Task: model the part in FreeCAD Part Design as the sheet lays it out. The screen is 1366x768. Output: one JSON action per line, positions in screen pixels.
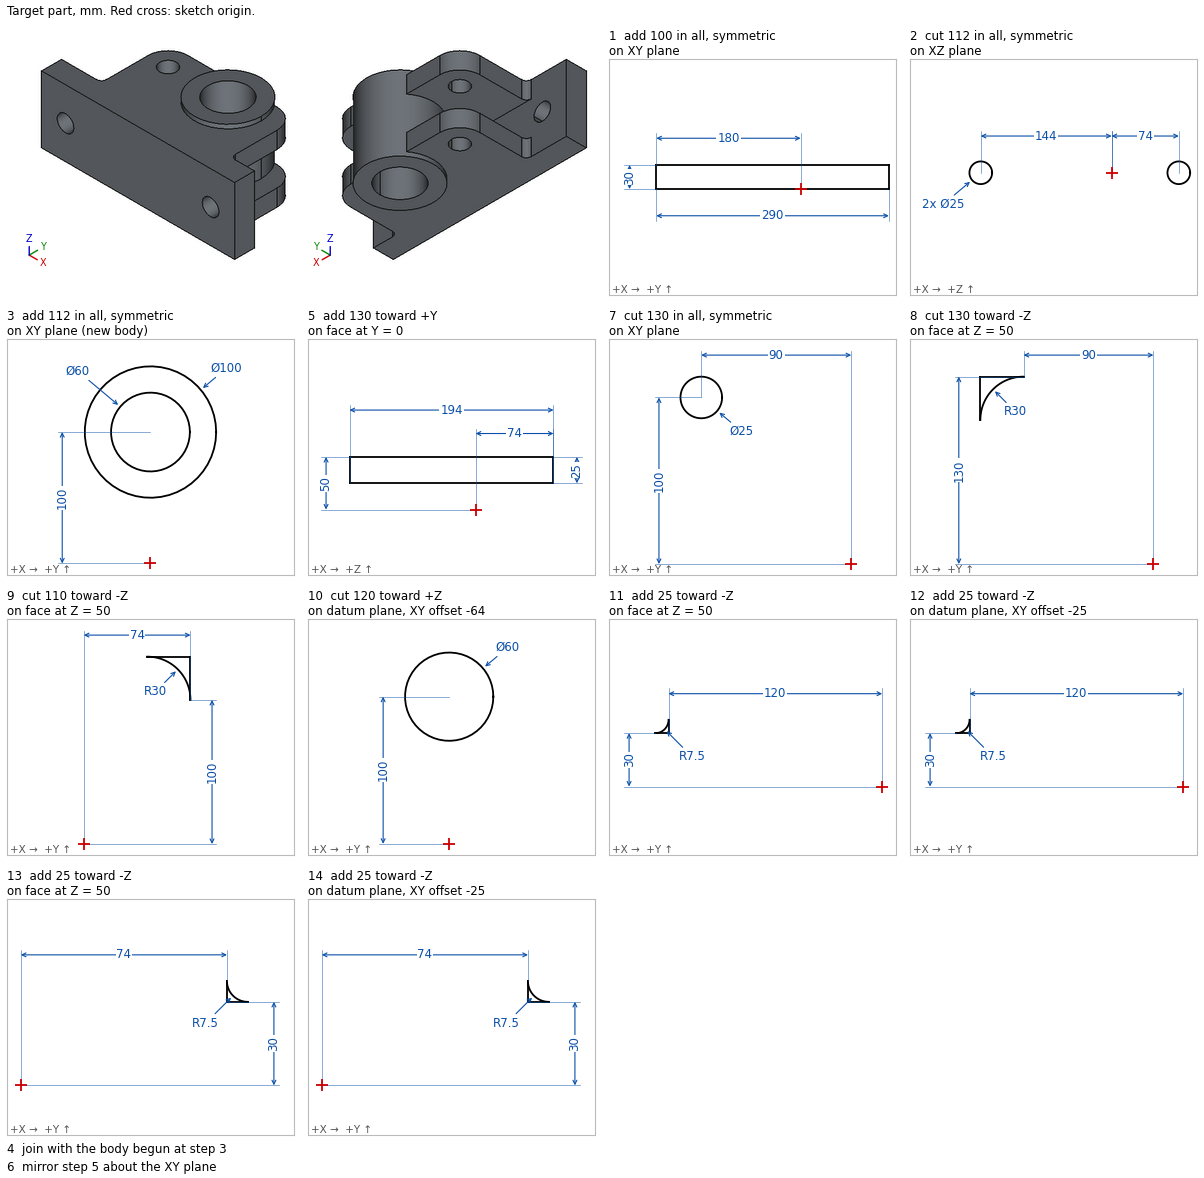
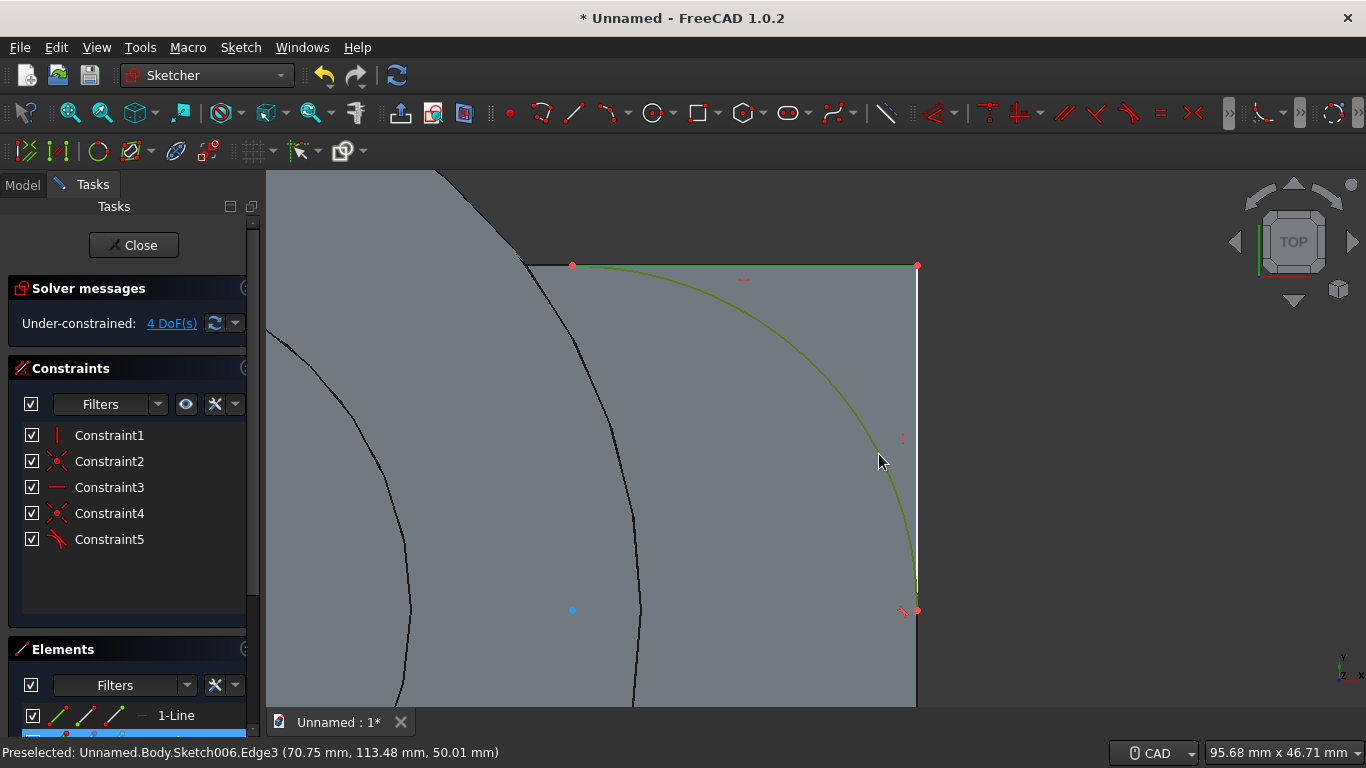
{"action": "left_click", "coordinate": [1130, 114]}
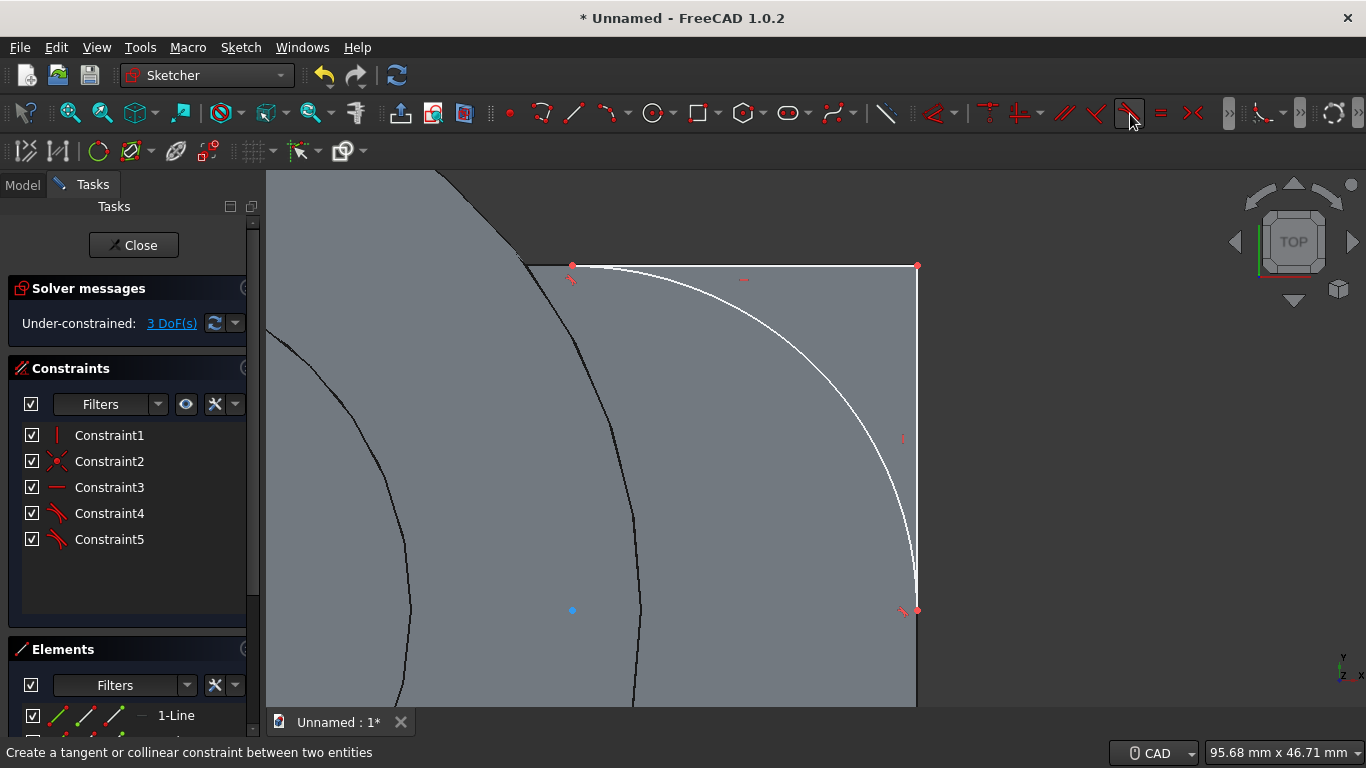
{"action": "left_click", "coordinate": [934, 114]}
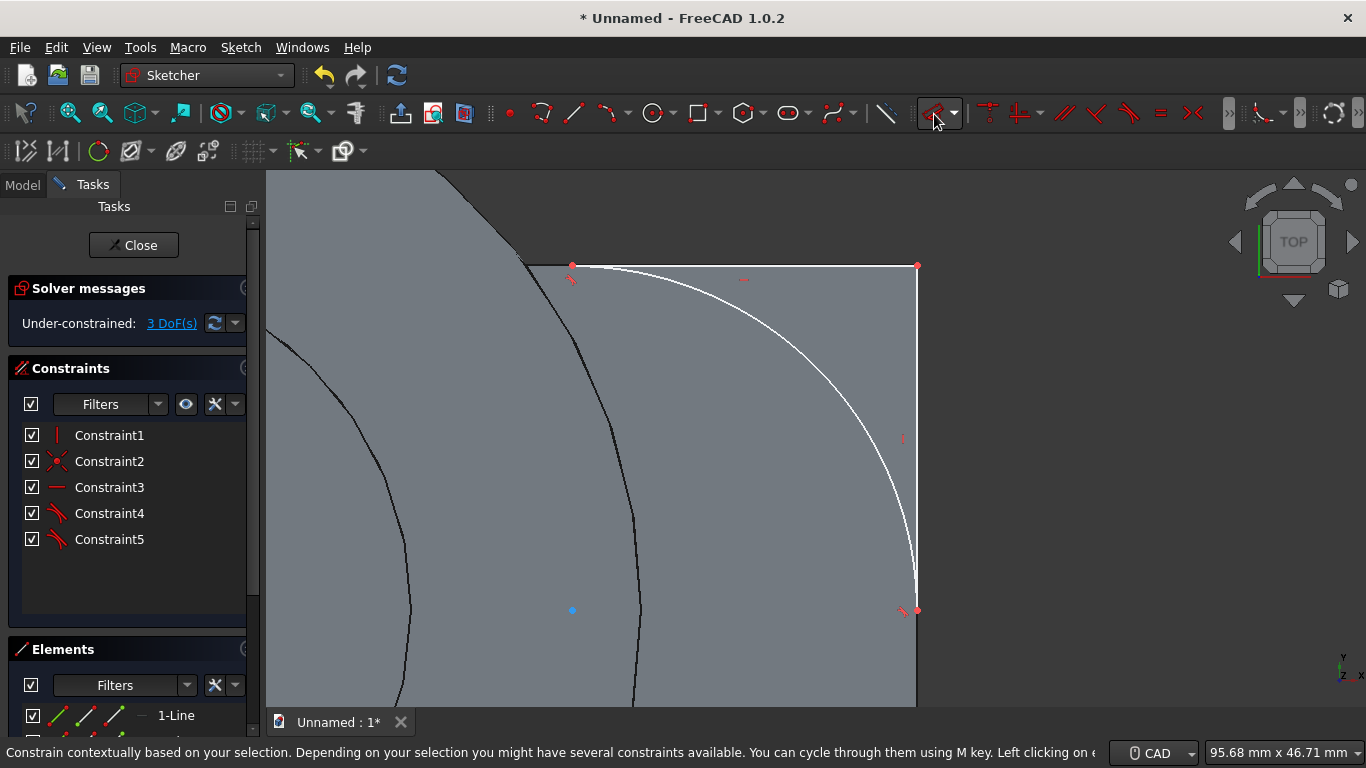
{"action": "left_click", "coordinate": [879, 454]}
{"action": "left_click", "coordinate": [949, 621]}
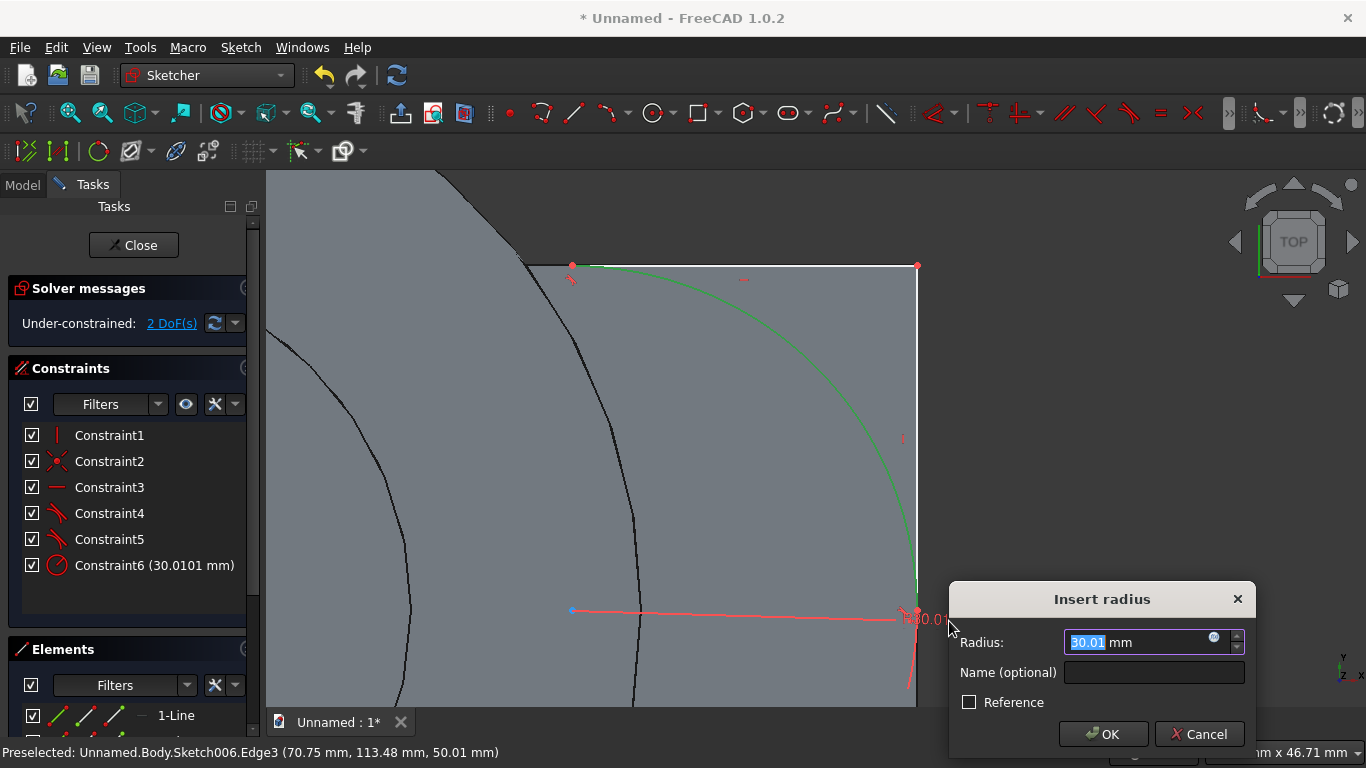
{"action": "type", "text": "30"}
{"action": "key", "text": "Return"}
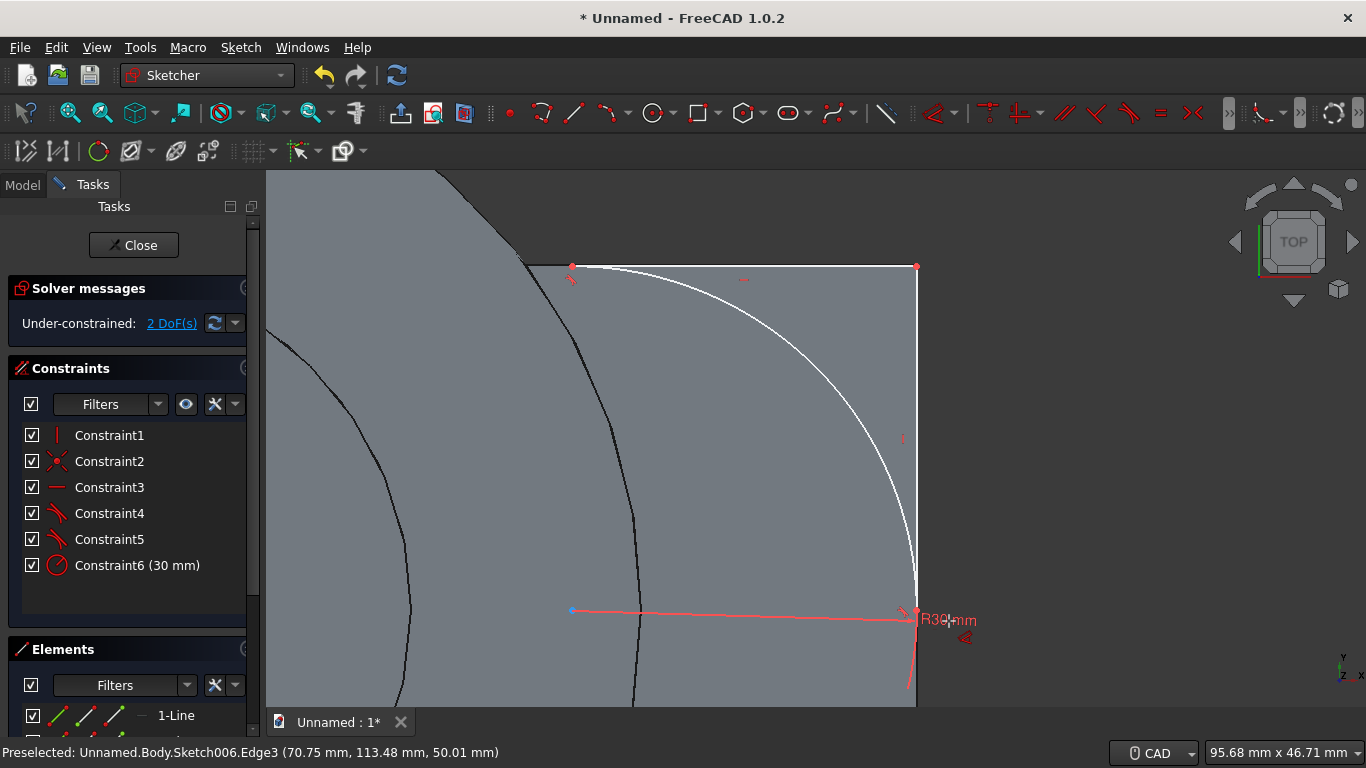
{"action": "left_click", "coordinate": [917, 611]}
{"action": "left_click", "coordinate": [605, 577]}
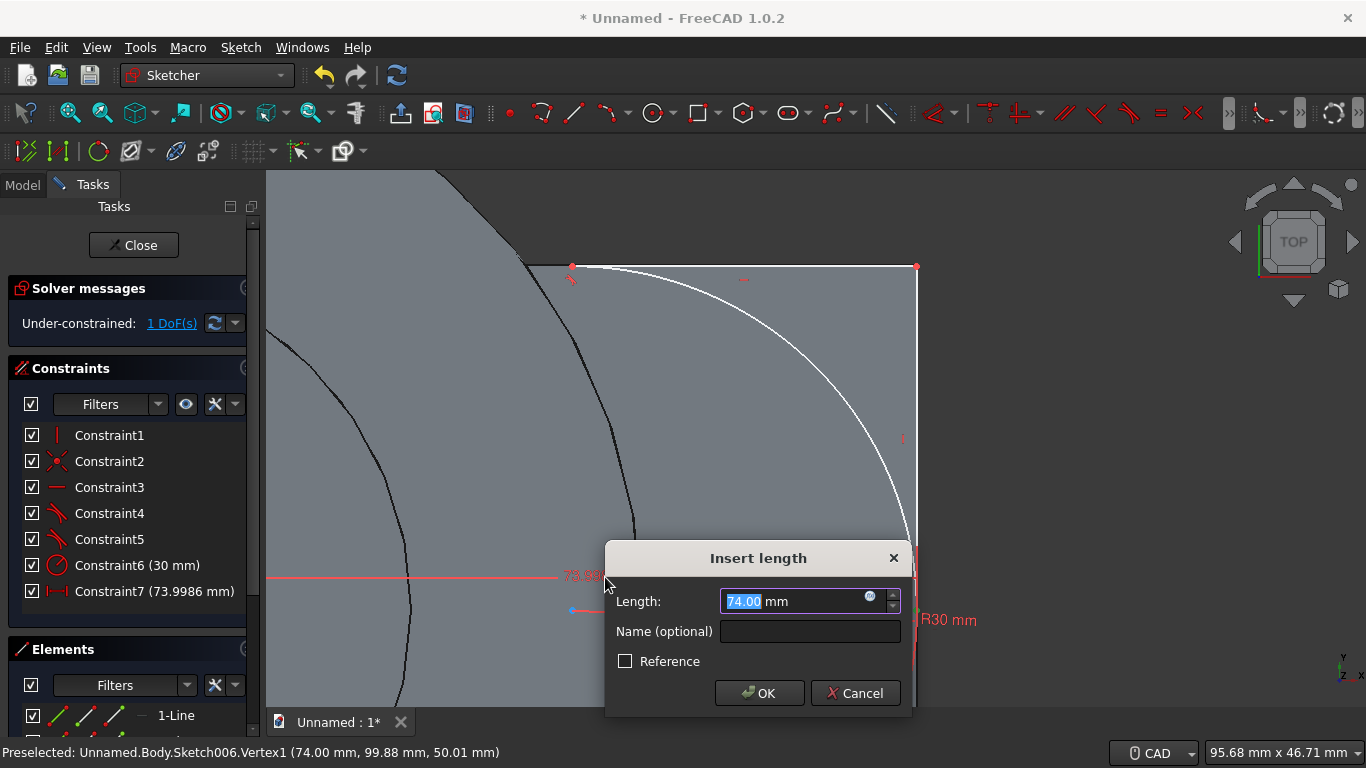
{"action": "type", "text": "74"}
{"action": "key", "text": "Return"}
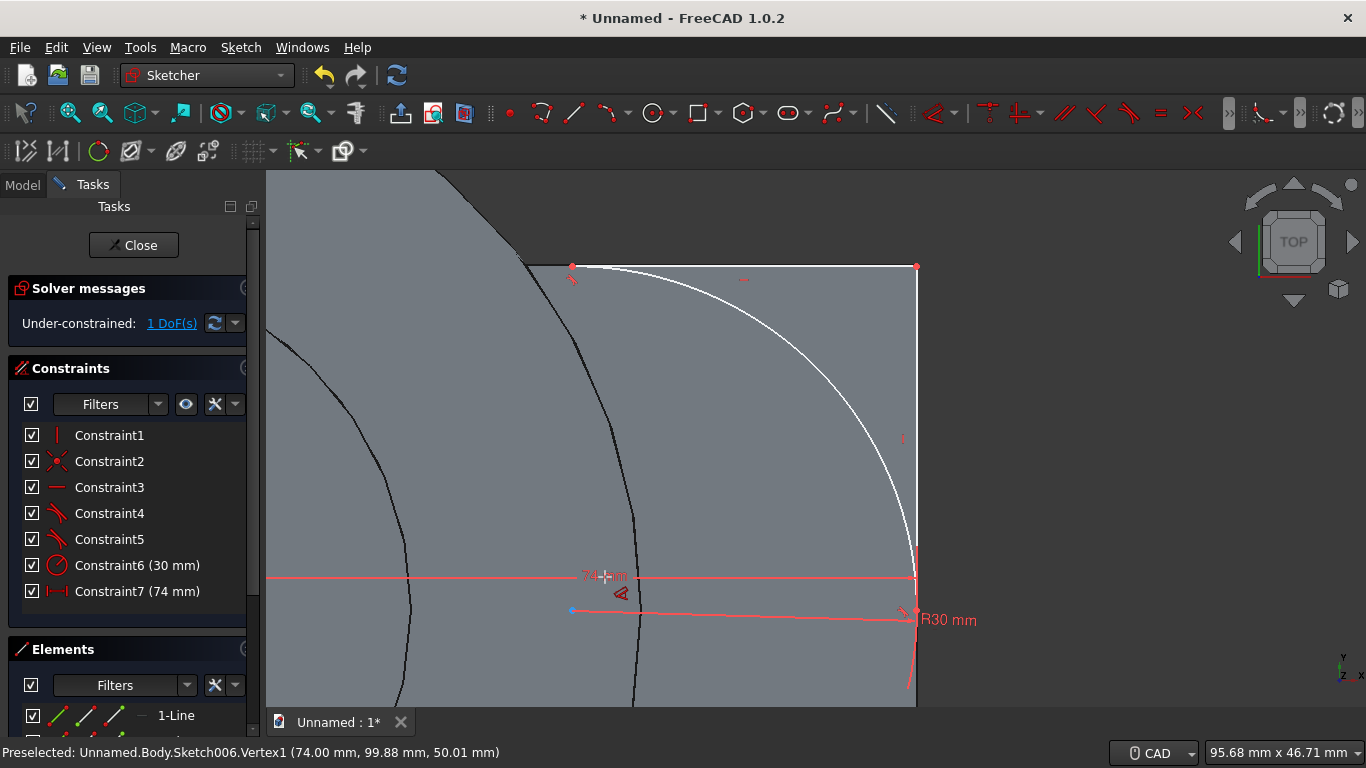
{"action": "left_click", "coordinate": [917, 611]}
{"action": "left_click", "coordinate": [951, 645]}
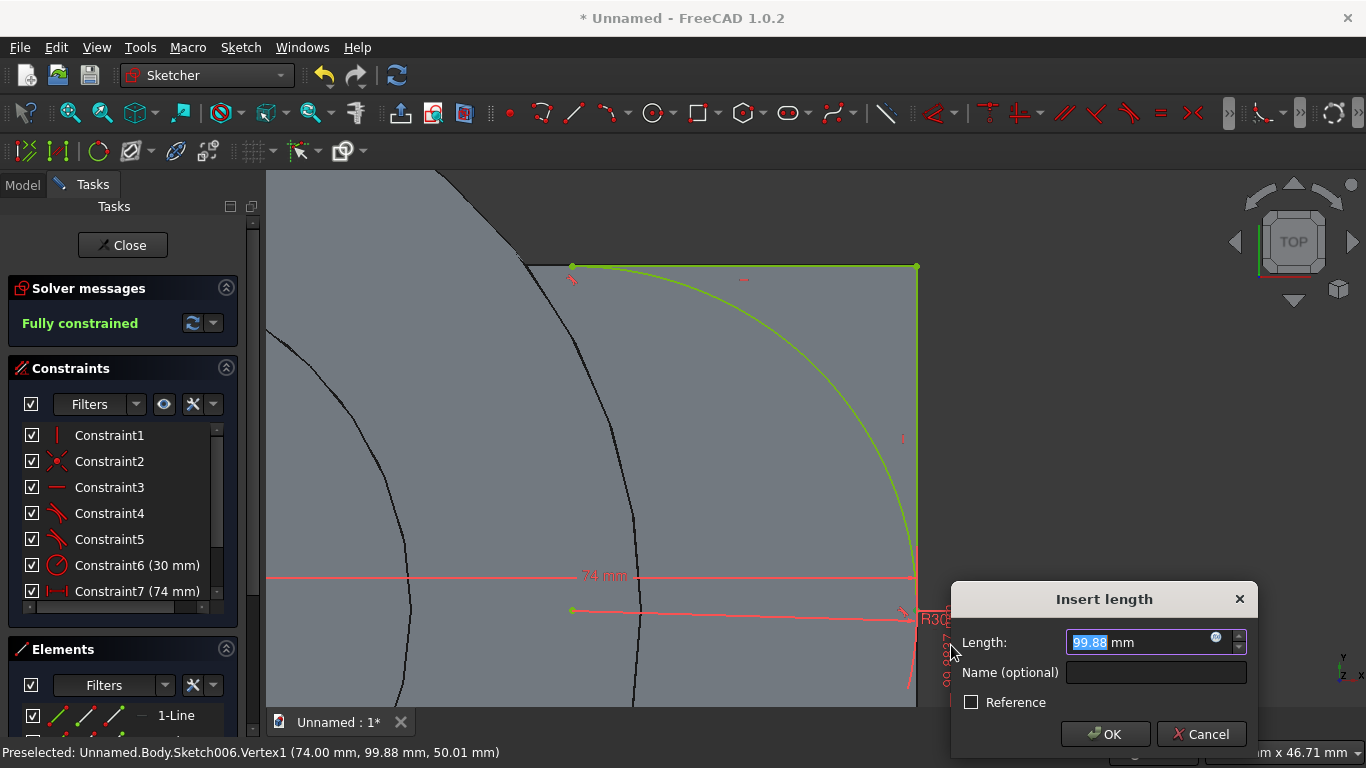
{"action": "type", "text": "100"}
{"action": "key", "text": "Return"}
{"action": "key", "text": "Escape"}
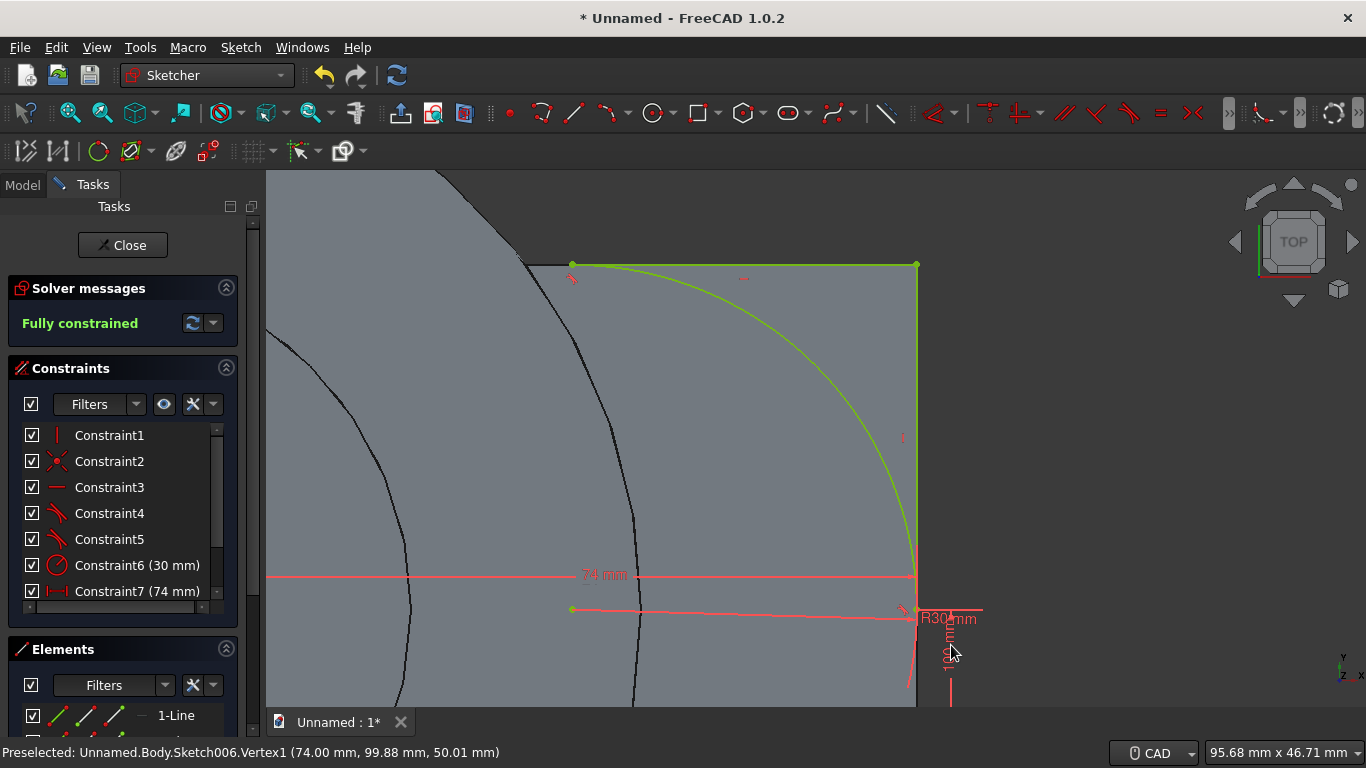
{"action": "left_click", "coordinate": [123, 245]}